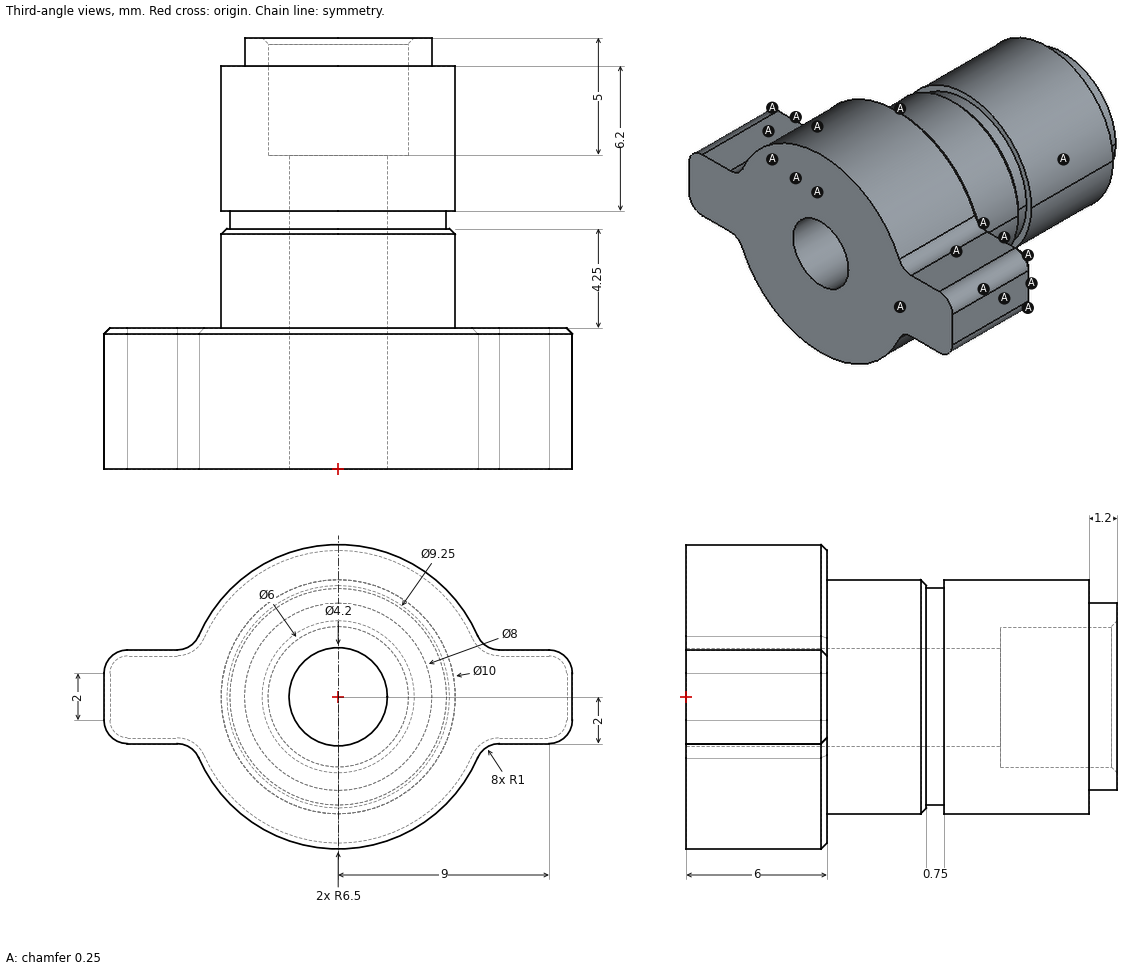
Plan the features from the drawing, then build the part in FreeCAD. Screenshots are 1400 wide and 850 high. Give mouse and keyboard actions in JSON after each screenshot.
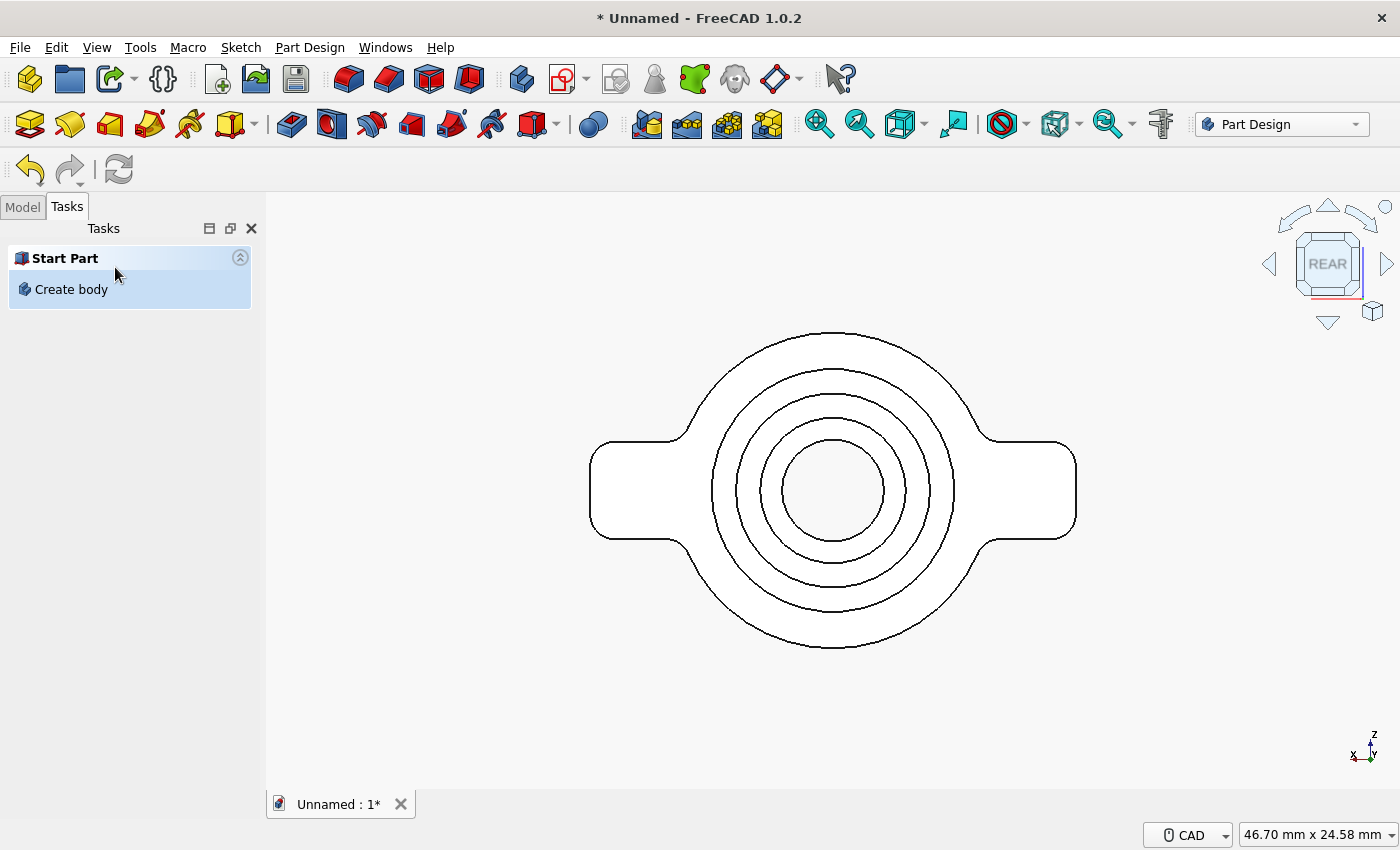
{"action": "left_click", "coordinate": [987, 542]}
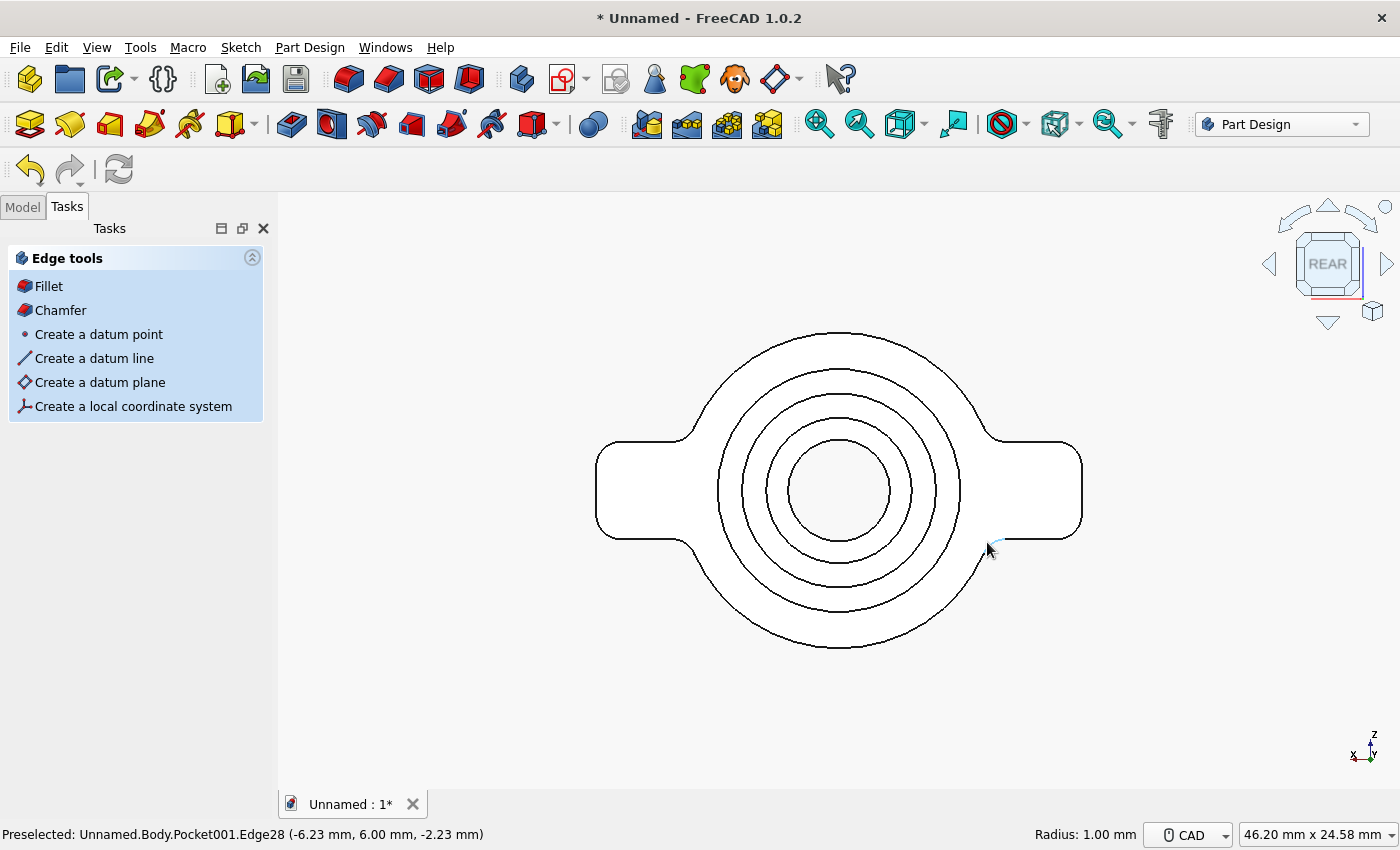
{"action": "left_click", "coordinate": [1032, 538], "text": "ctrl"}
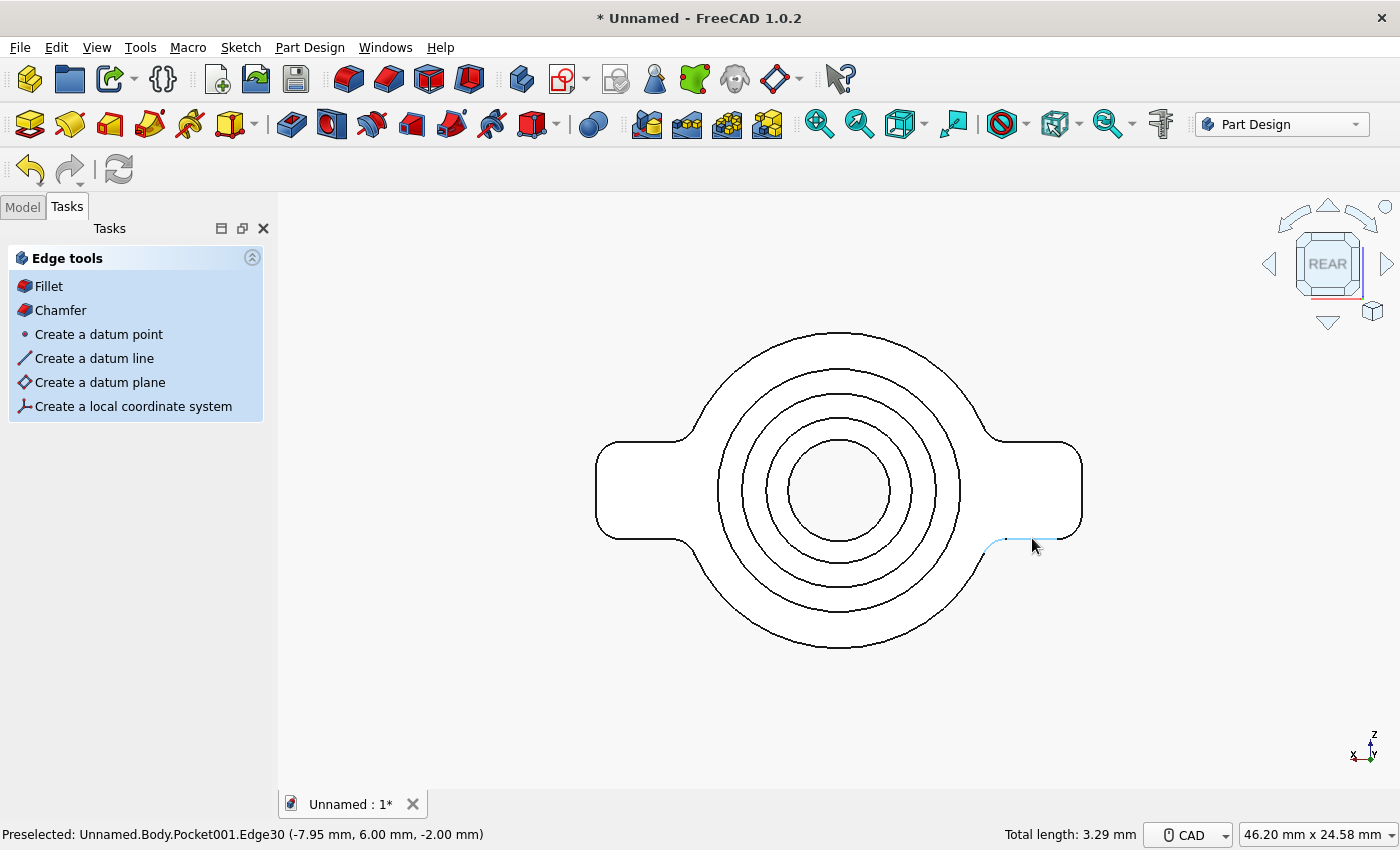
{"action": "left_click", "coordinate": [1075, 531], "text": "ctrl"}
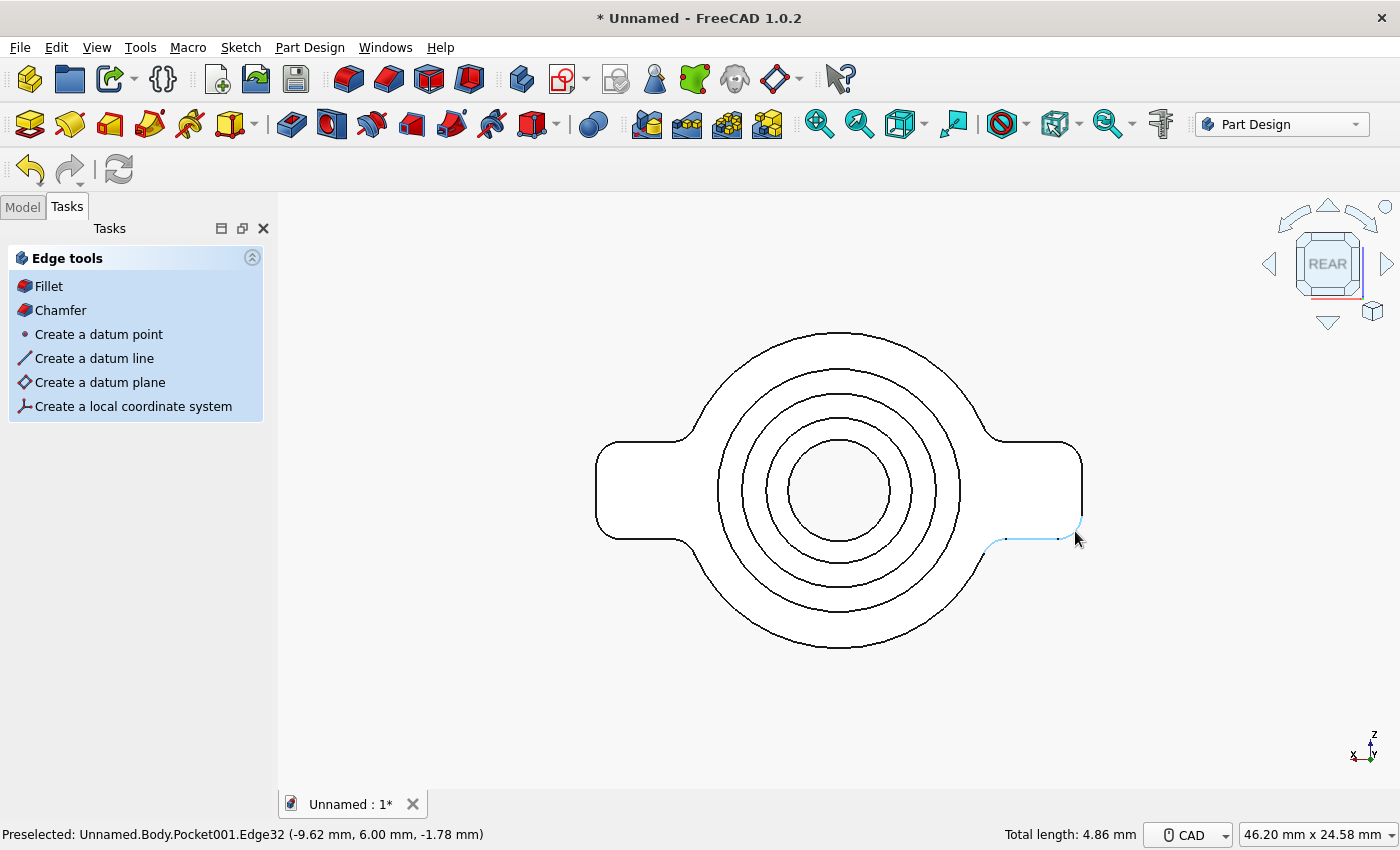
{"action": "left_click", "coordinate": [1082, 490], "text": "ctrl"}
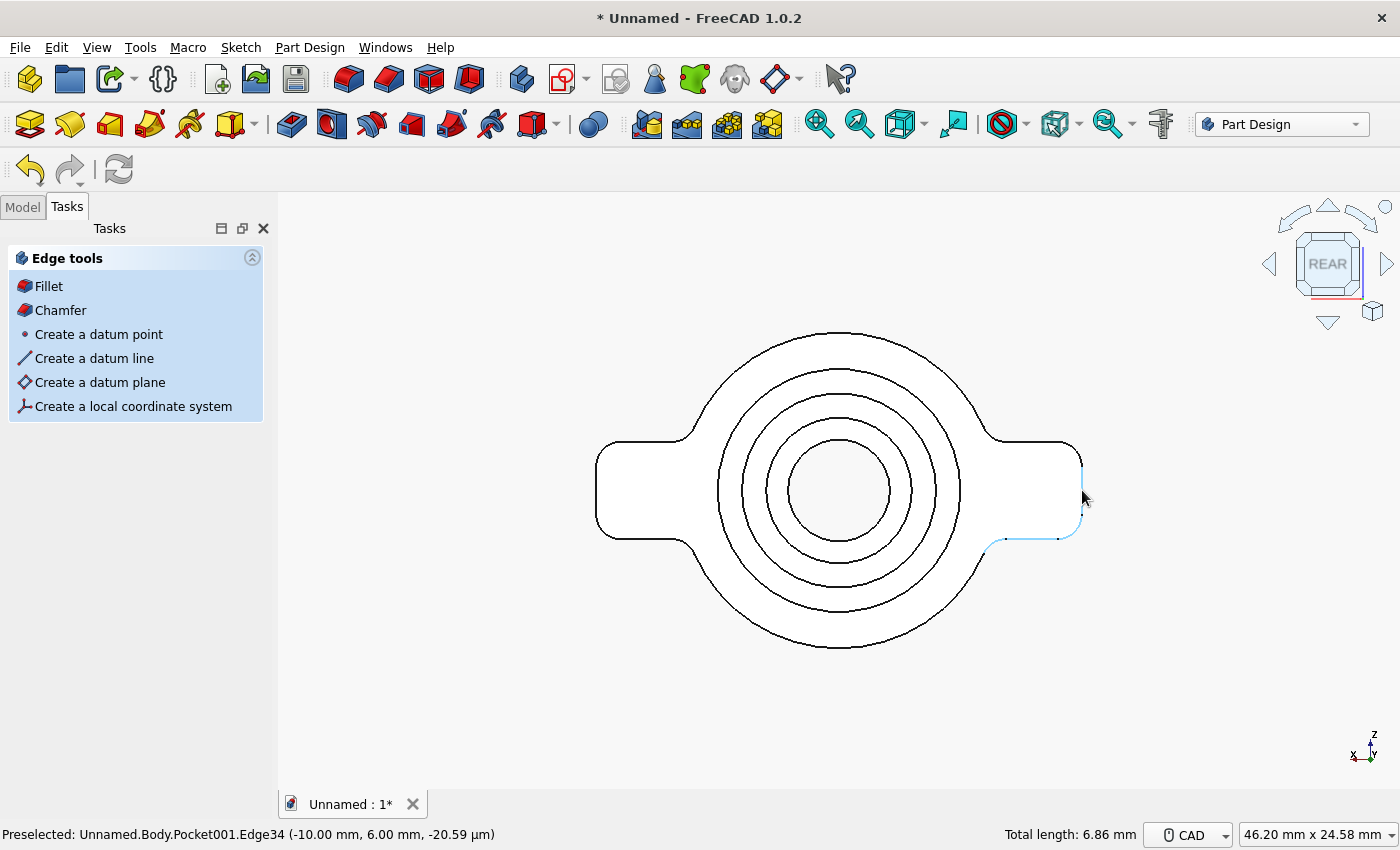
{"action": "left_click", "coordinate": [1075, 448], "text": "ctrl"}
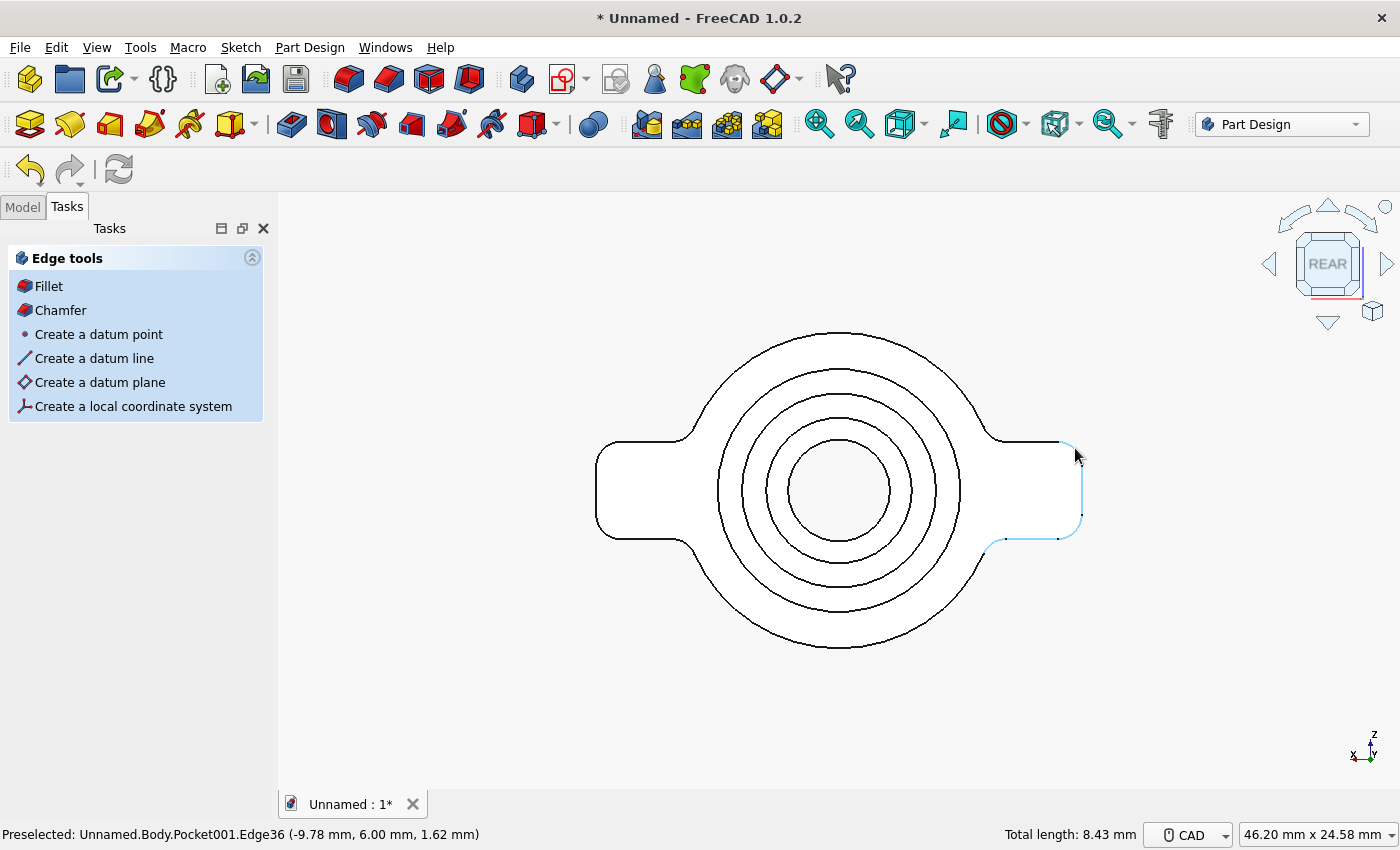
{"action": "left_click", "coordinate": [993, 437], "text": "ctrl"}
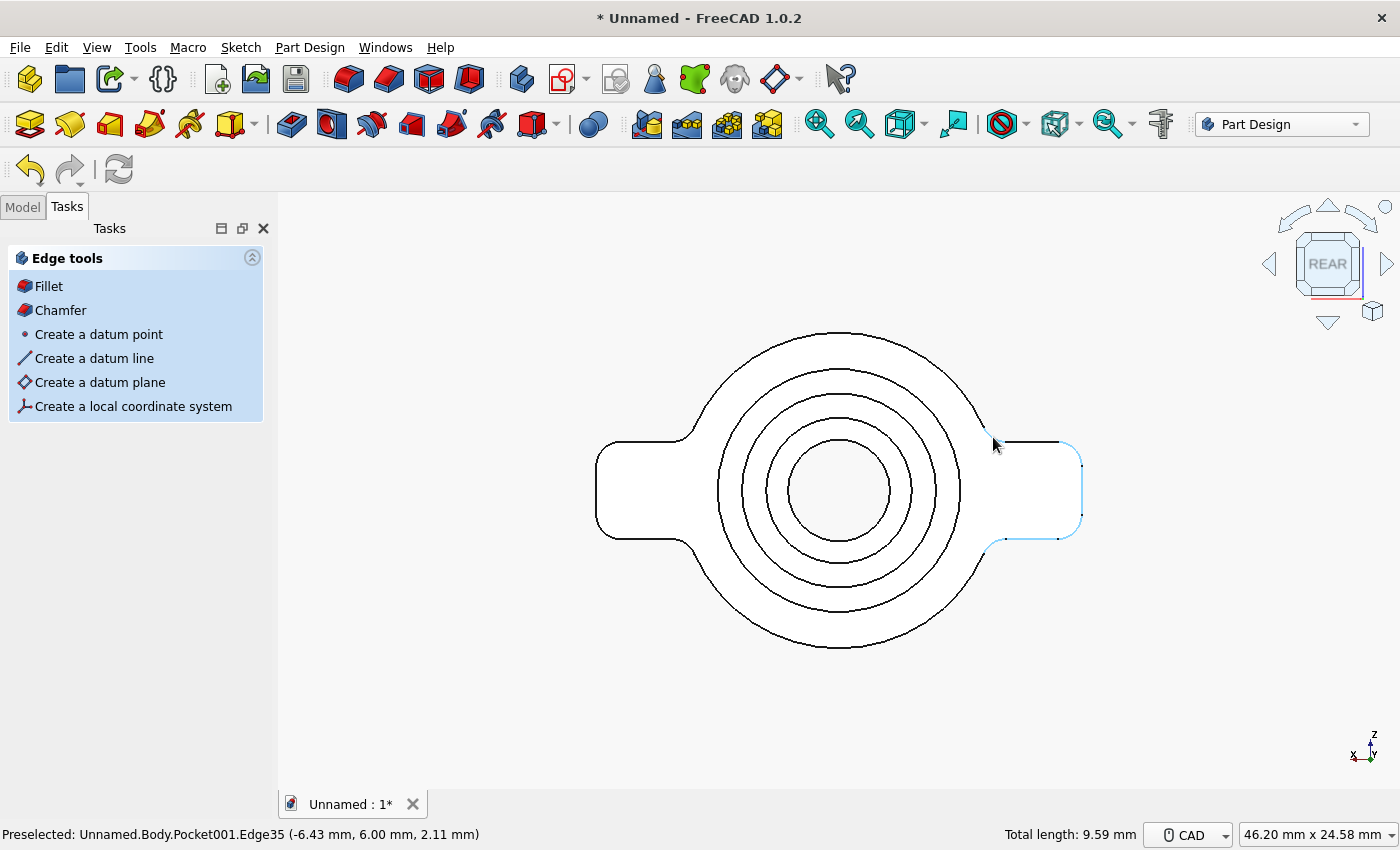
{"action": "left_click", "coordinate": [685, 542], "text": "ctrl"}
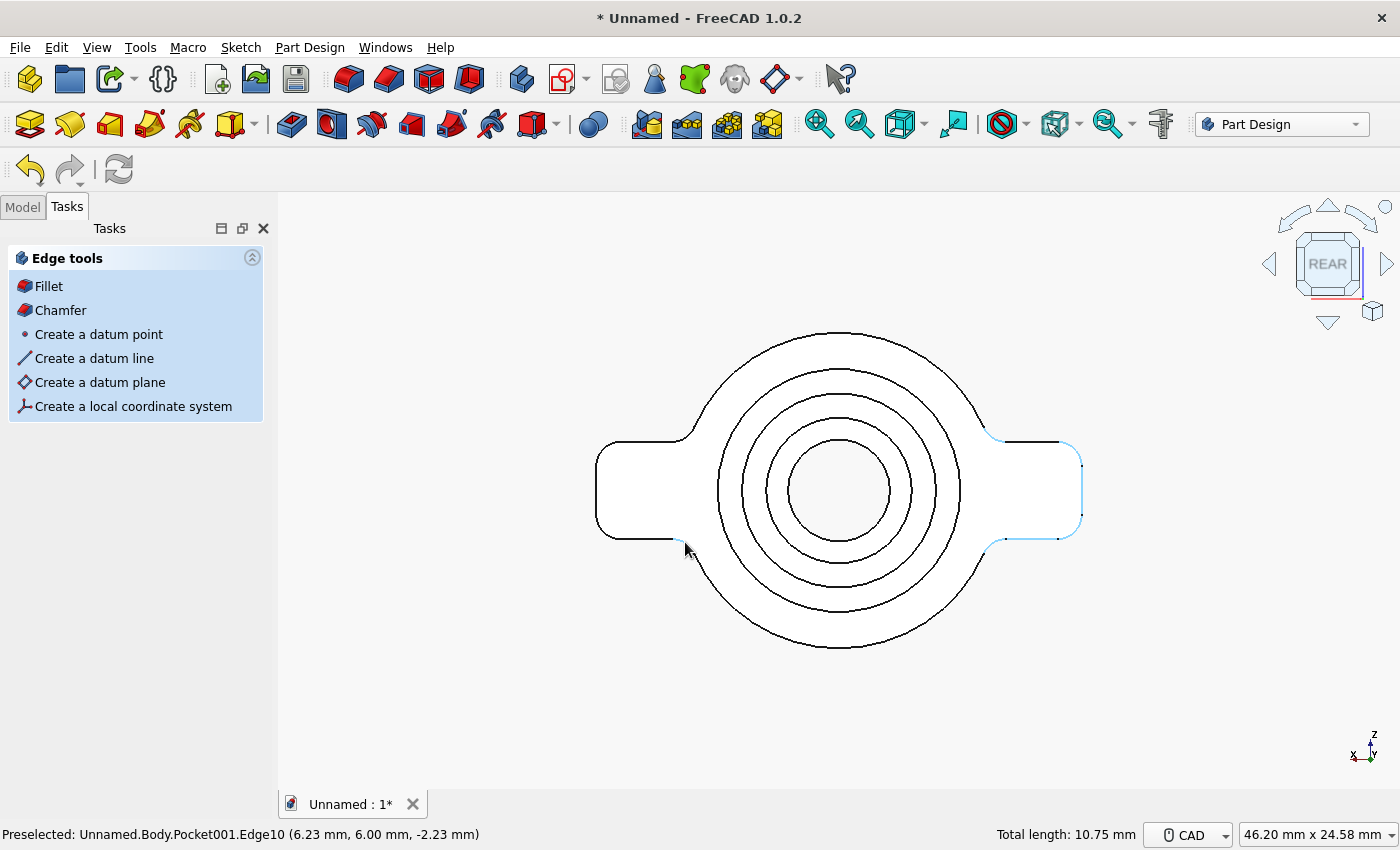
{"action": "left_click", "coordinate": [597, 458], "text": "ctrl"}